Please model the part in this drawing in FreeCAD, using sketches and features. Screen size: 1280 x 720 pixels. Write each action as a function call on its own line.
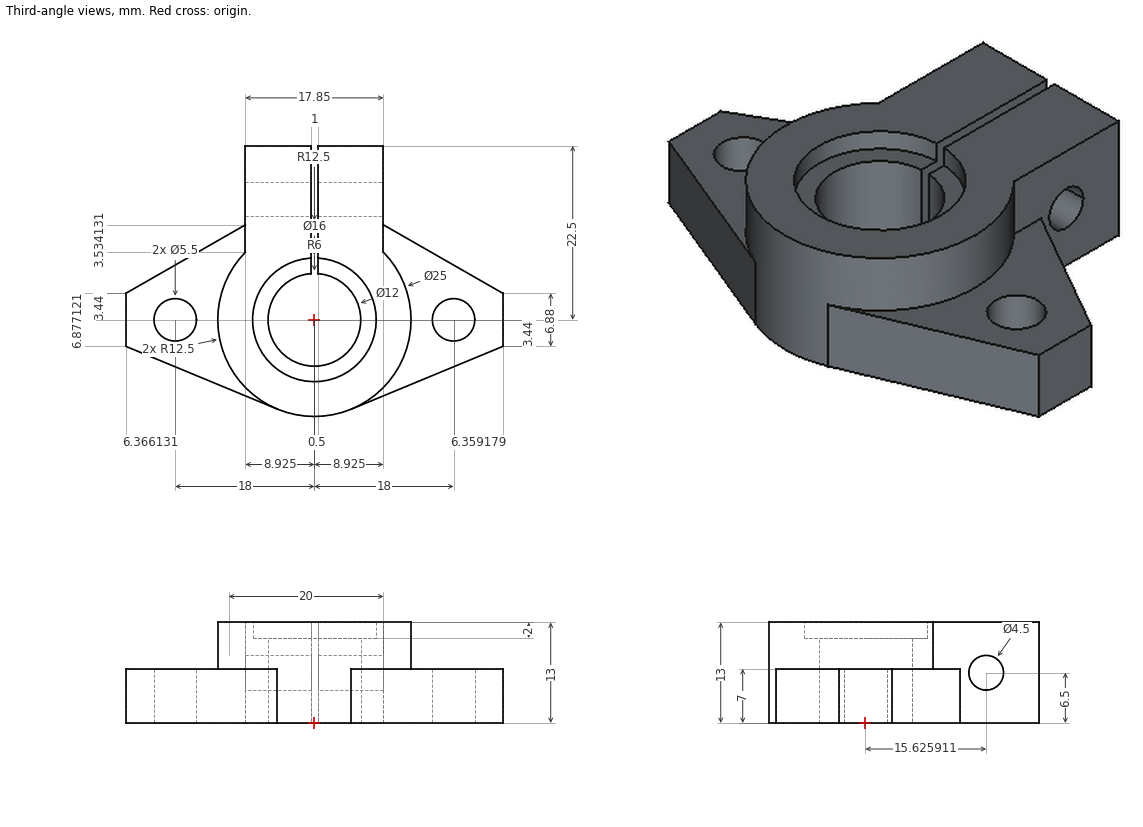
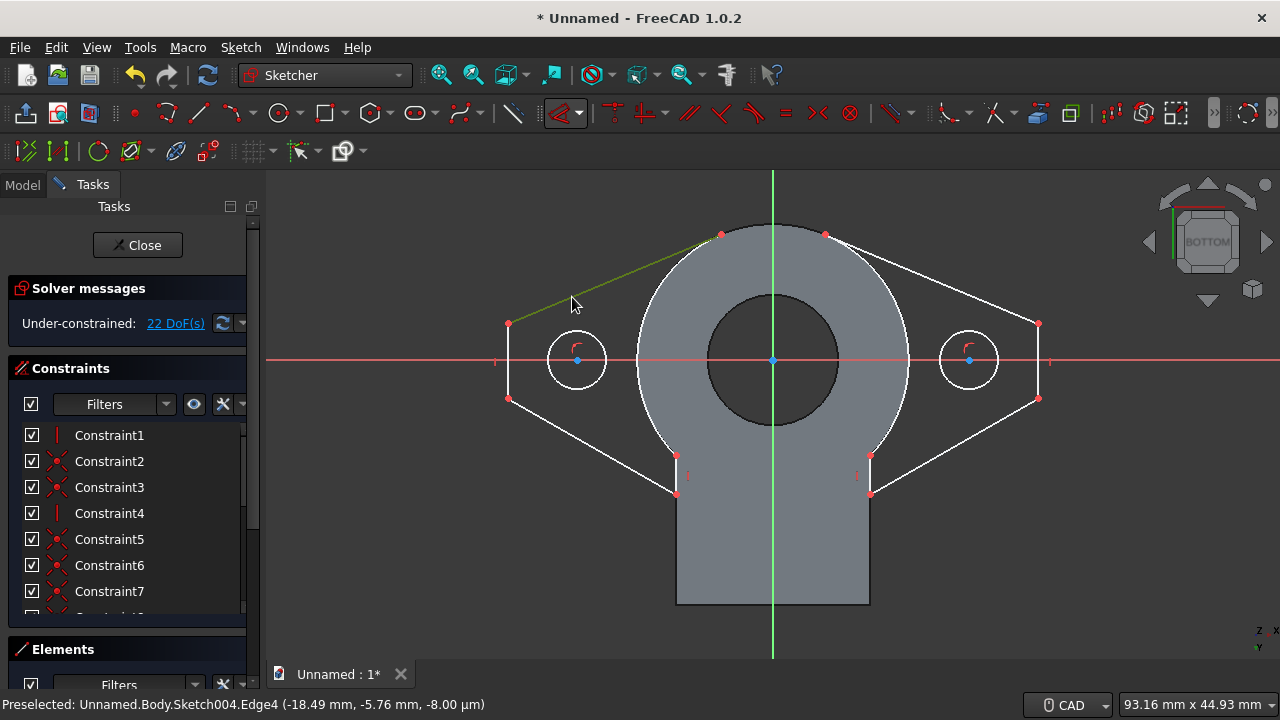
click(660, 285)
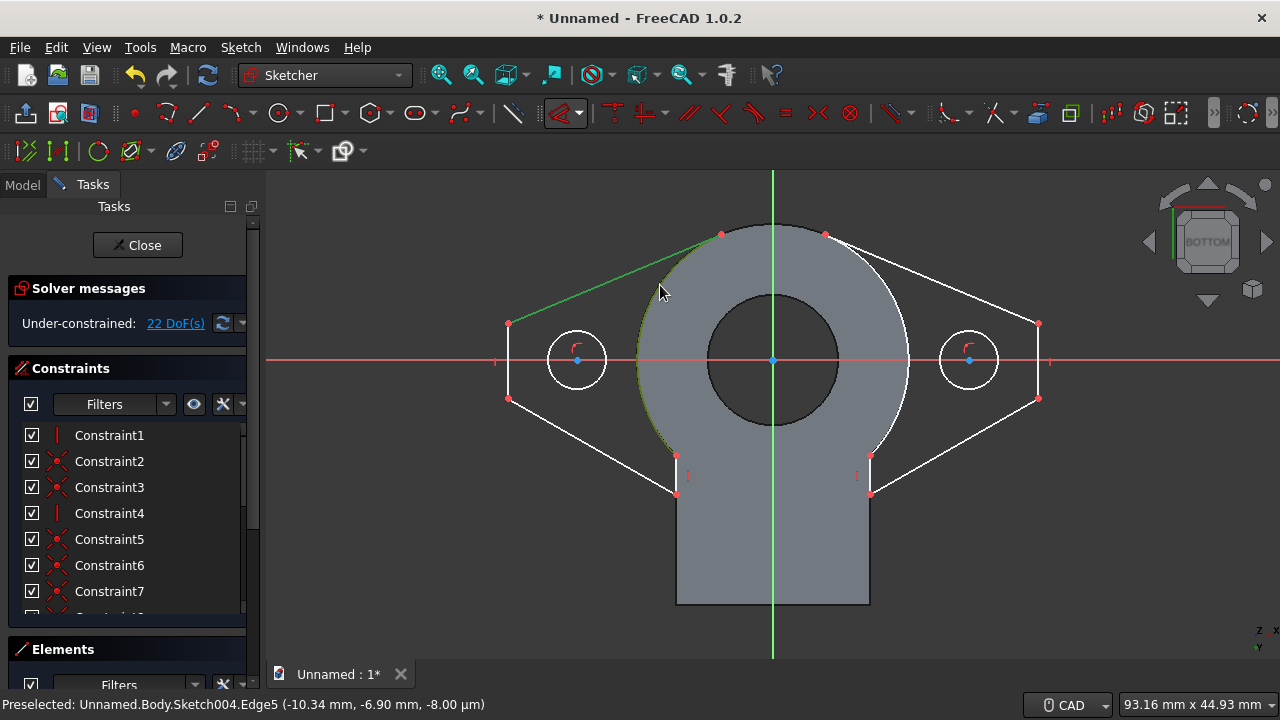
click(754, 114)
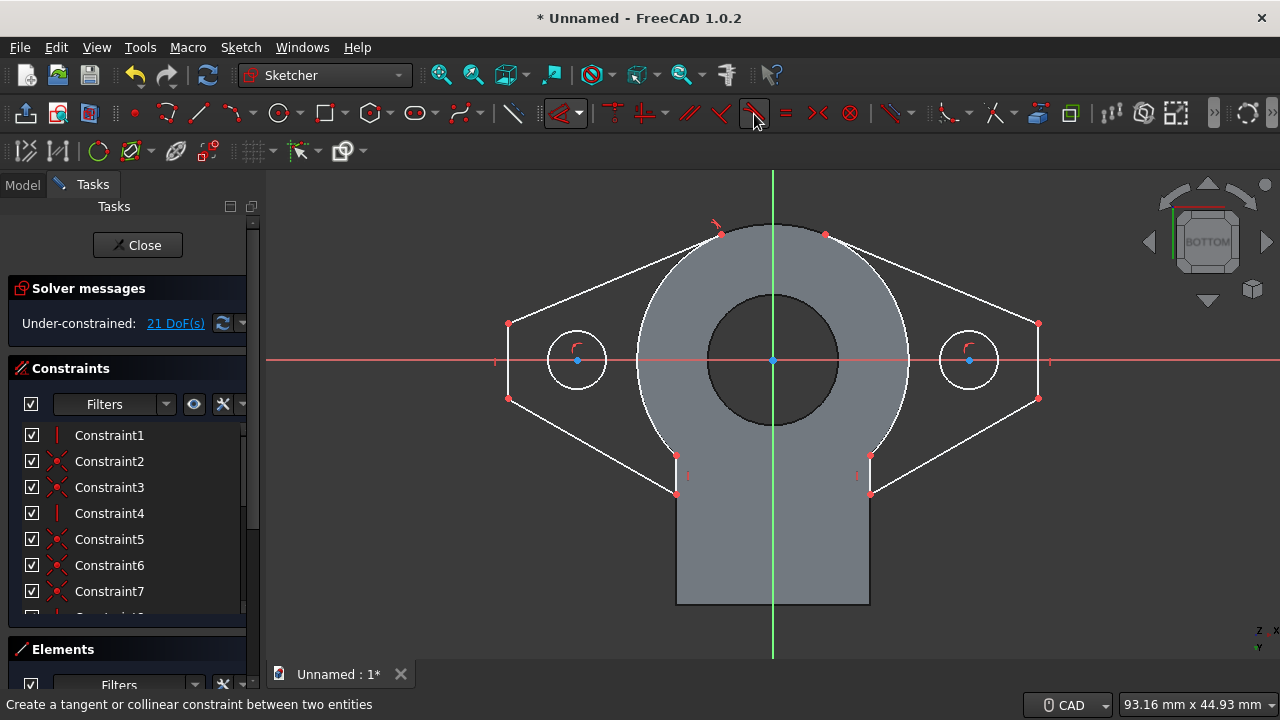
click(889, 262)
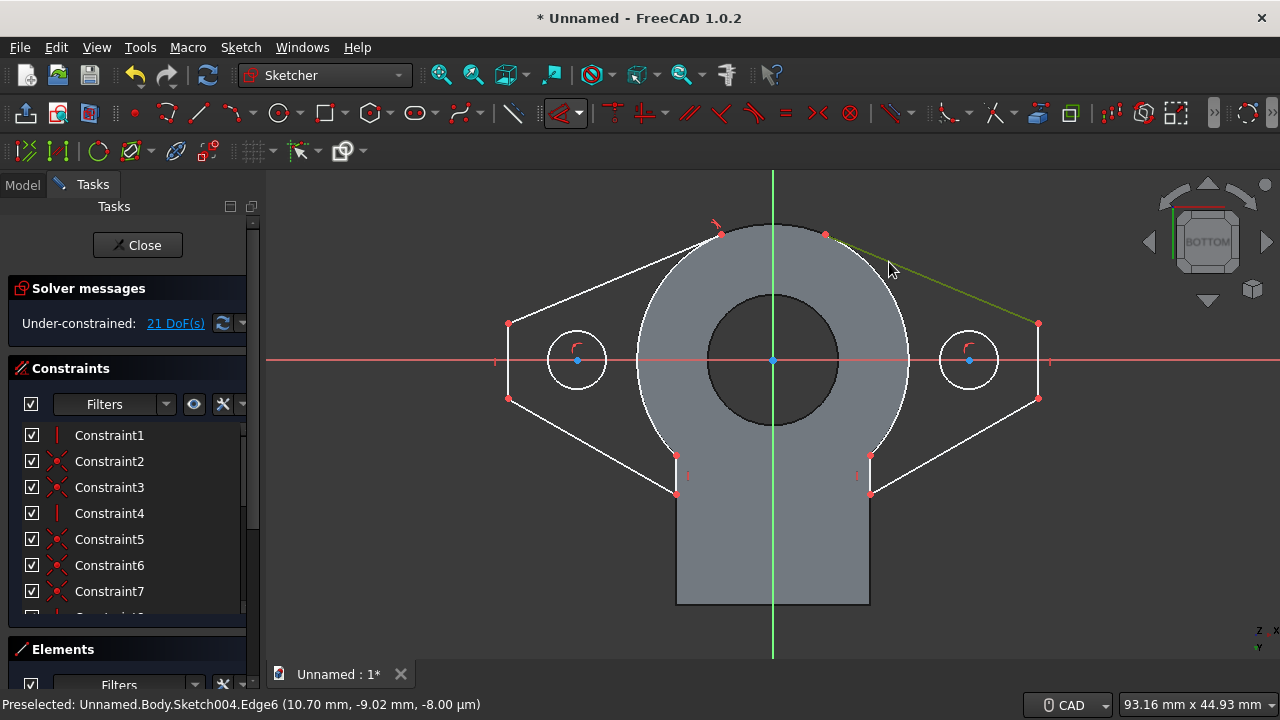
click(906, 386)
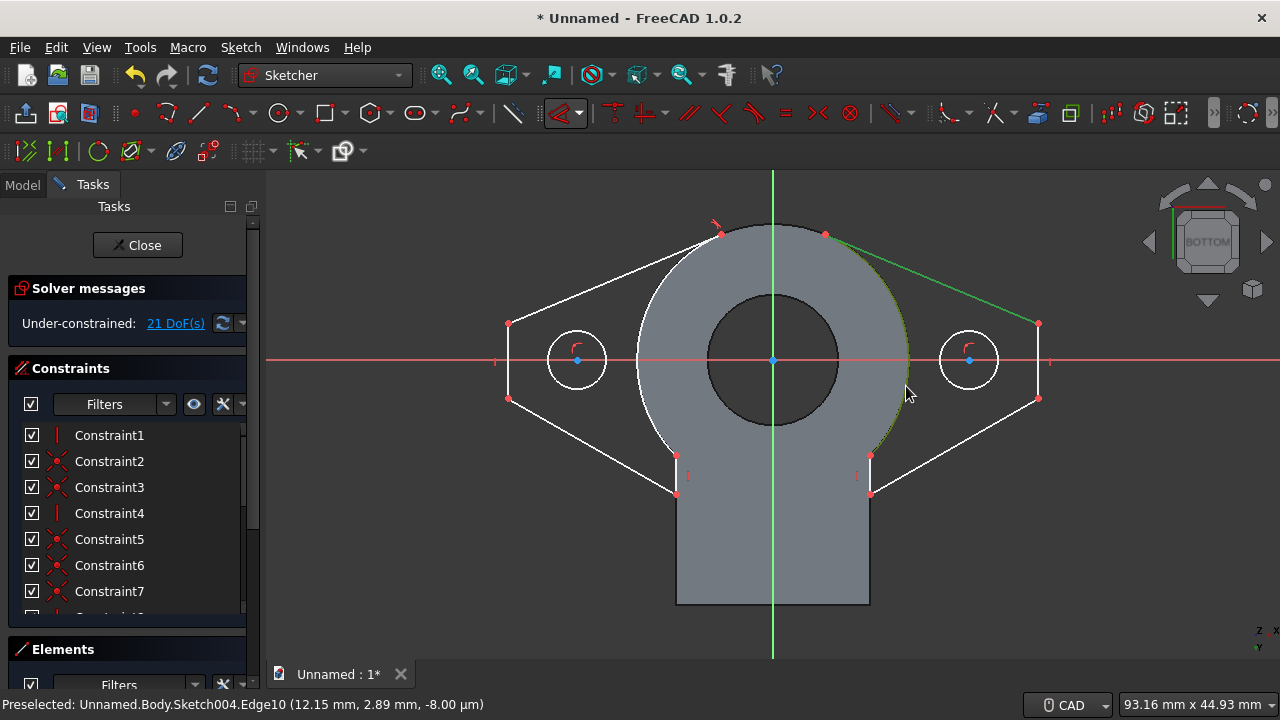
click(754, 114)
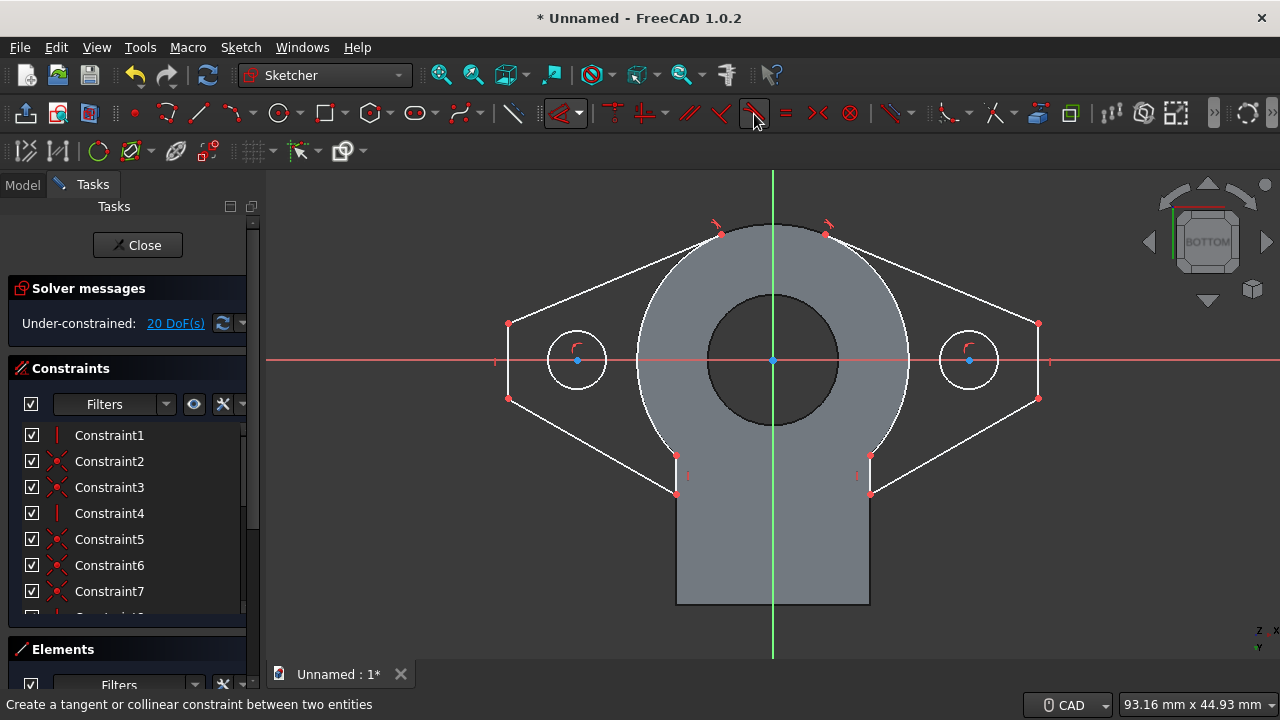
click(660, 285)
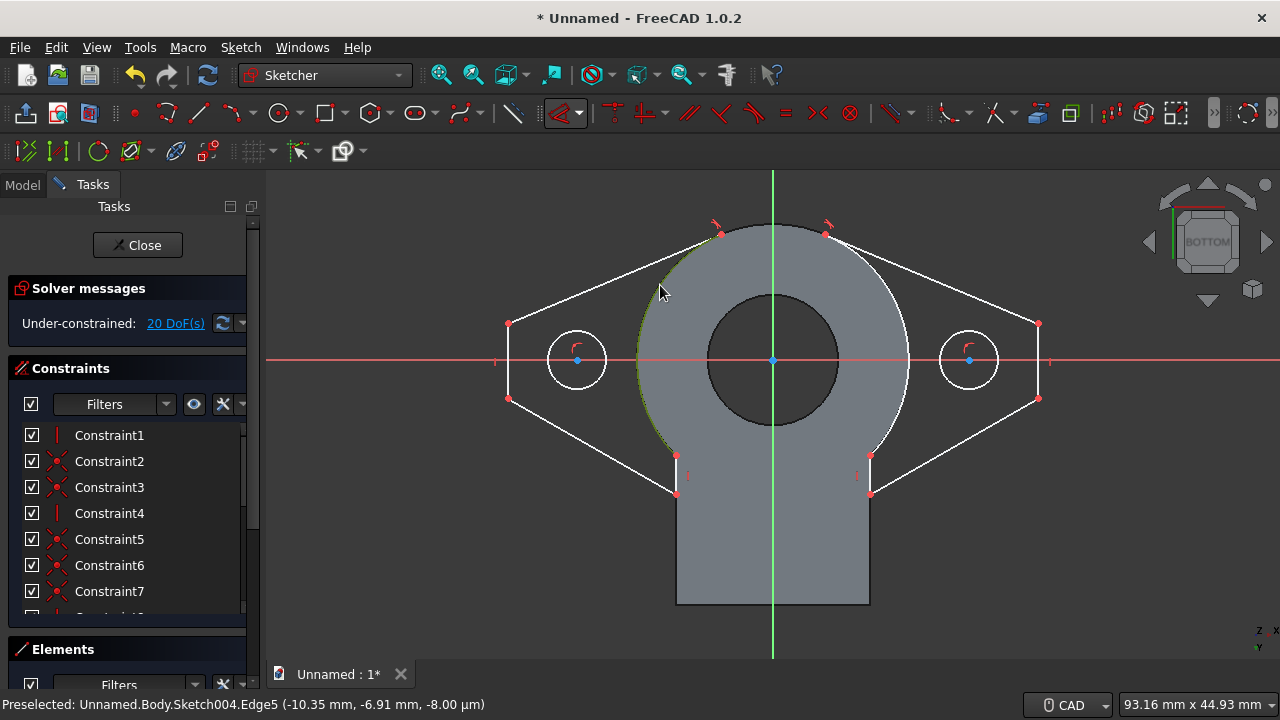
click(906, 386)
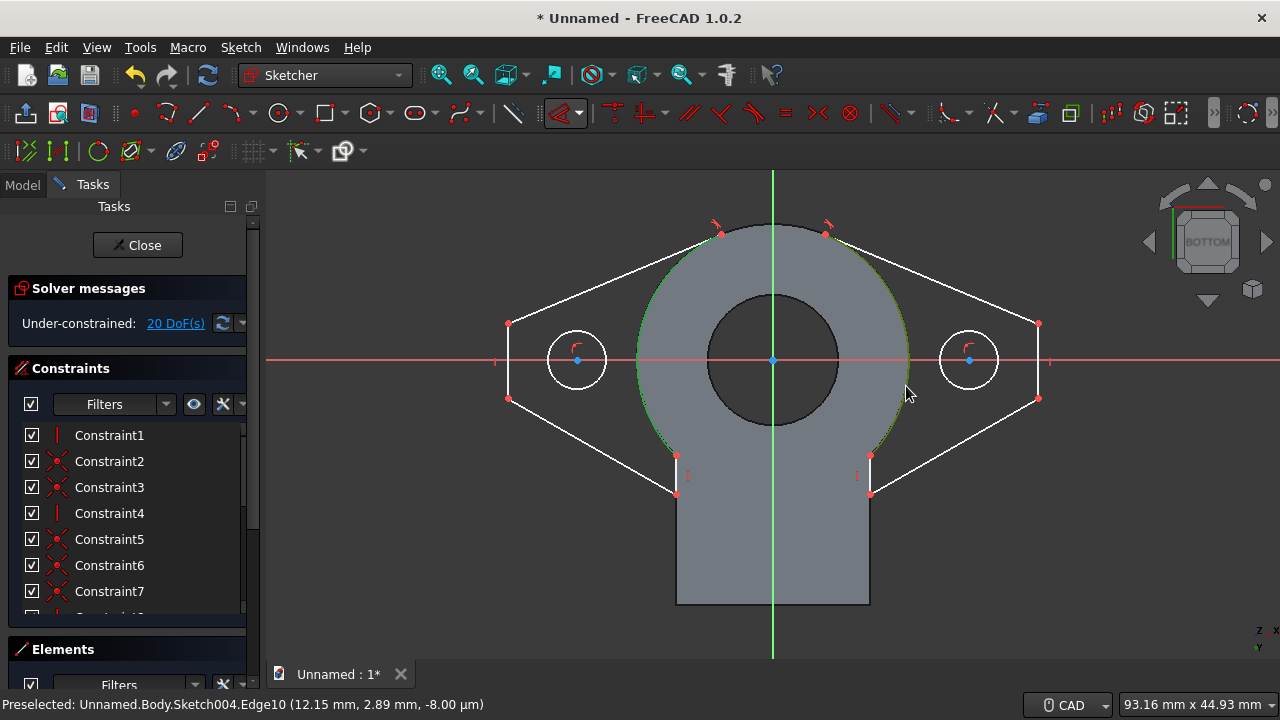
click(614, 114)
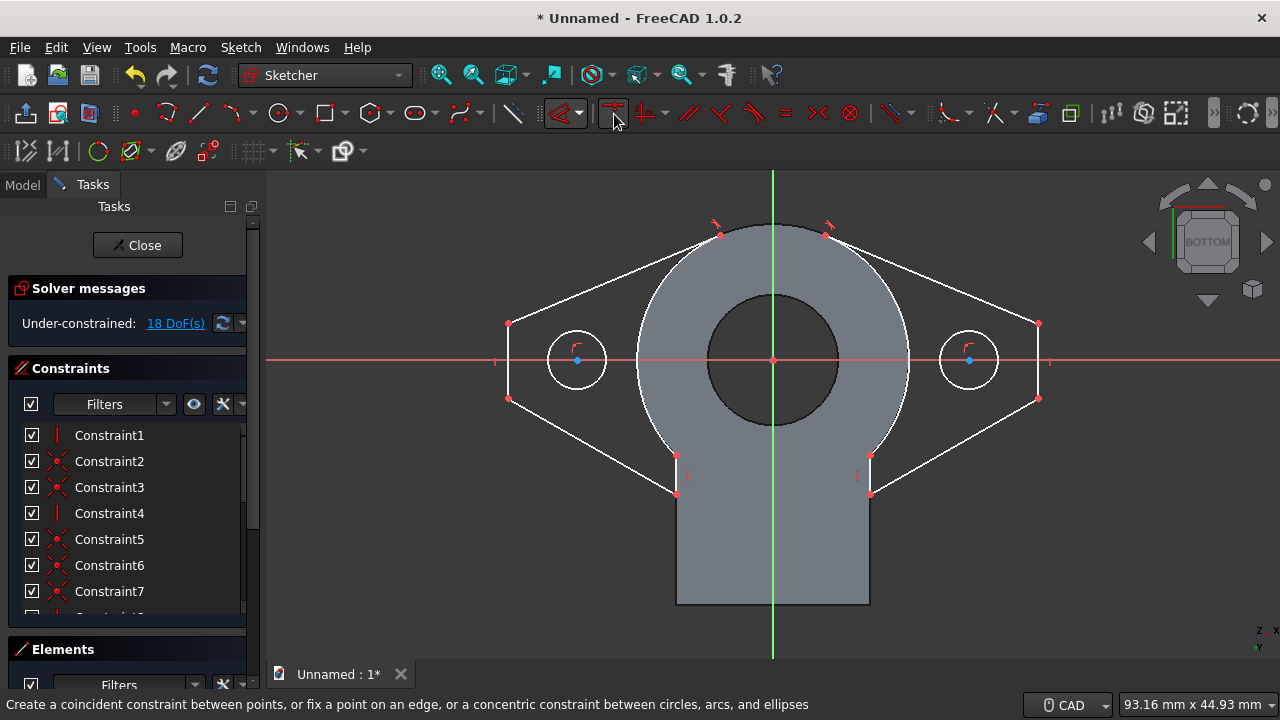
scroll(773, 360, up, 2)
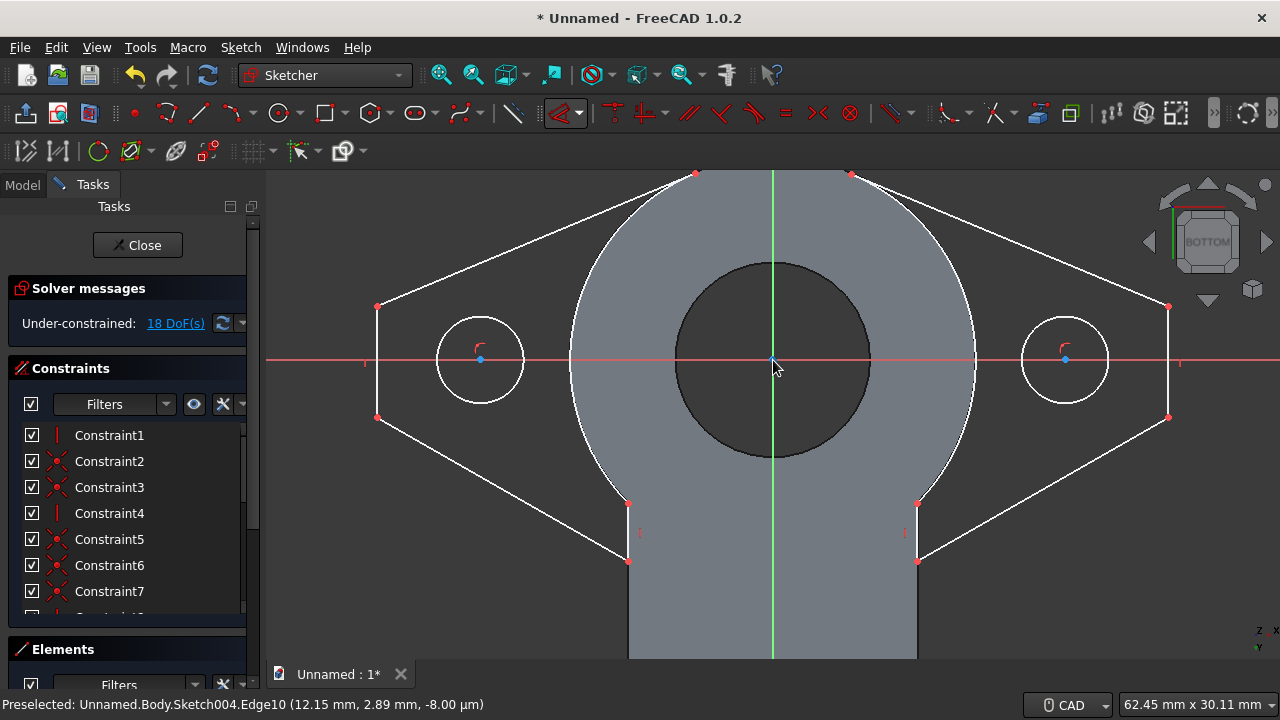
drag(763, 350, 783, 371)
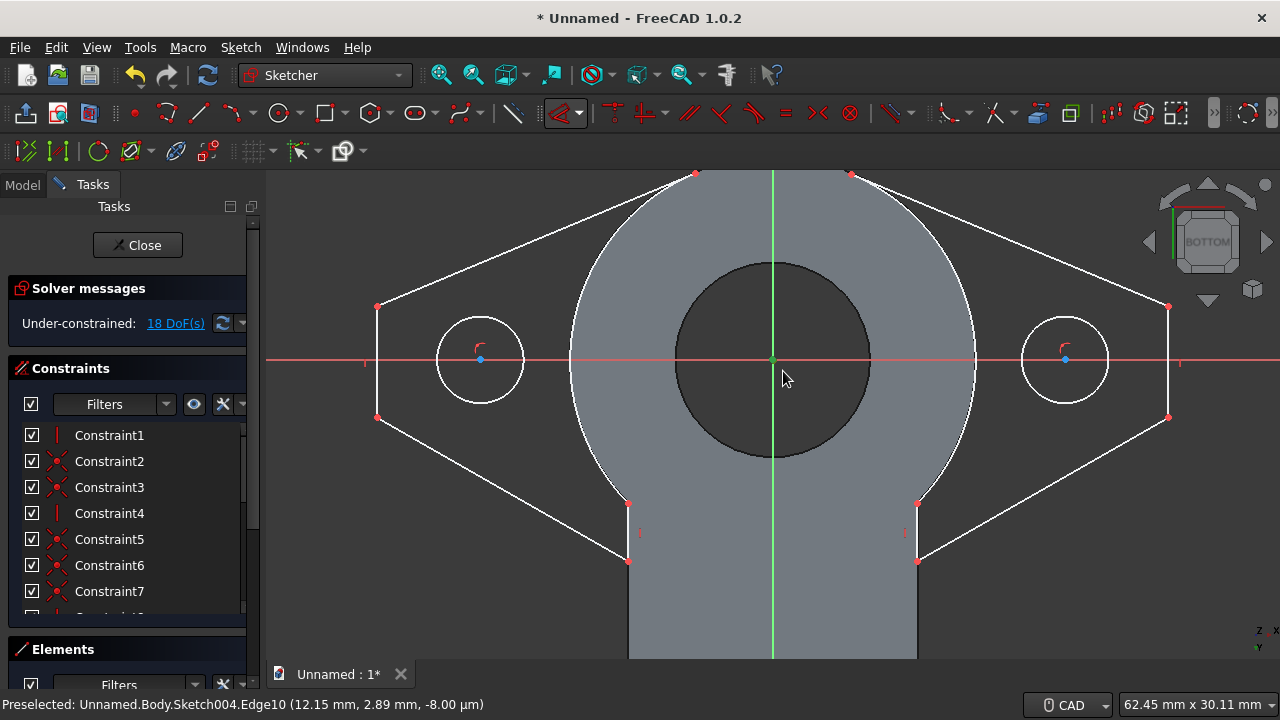
click(614, 114)